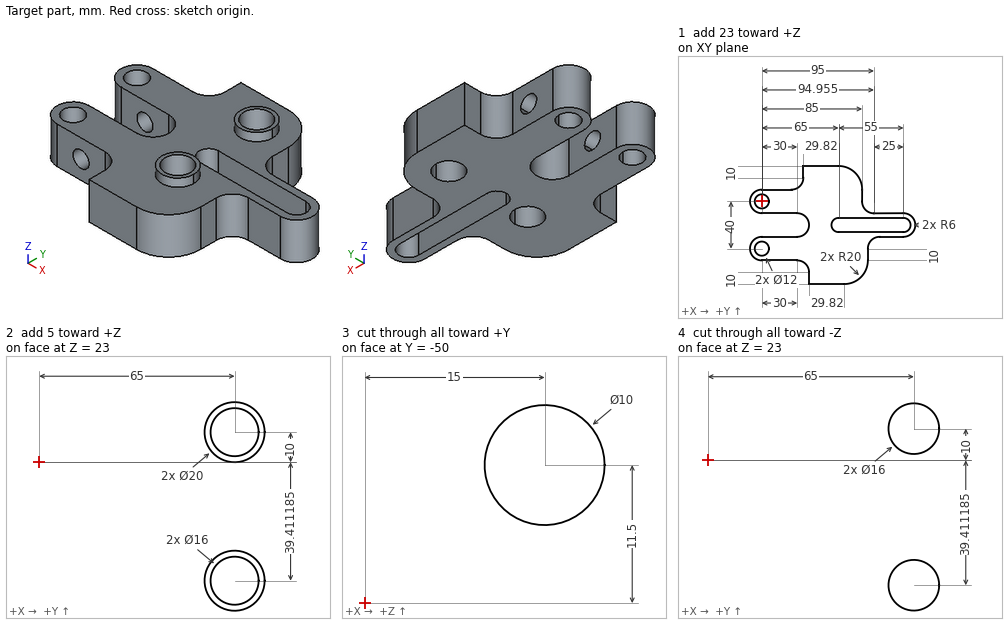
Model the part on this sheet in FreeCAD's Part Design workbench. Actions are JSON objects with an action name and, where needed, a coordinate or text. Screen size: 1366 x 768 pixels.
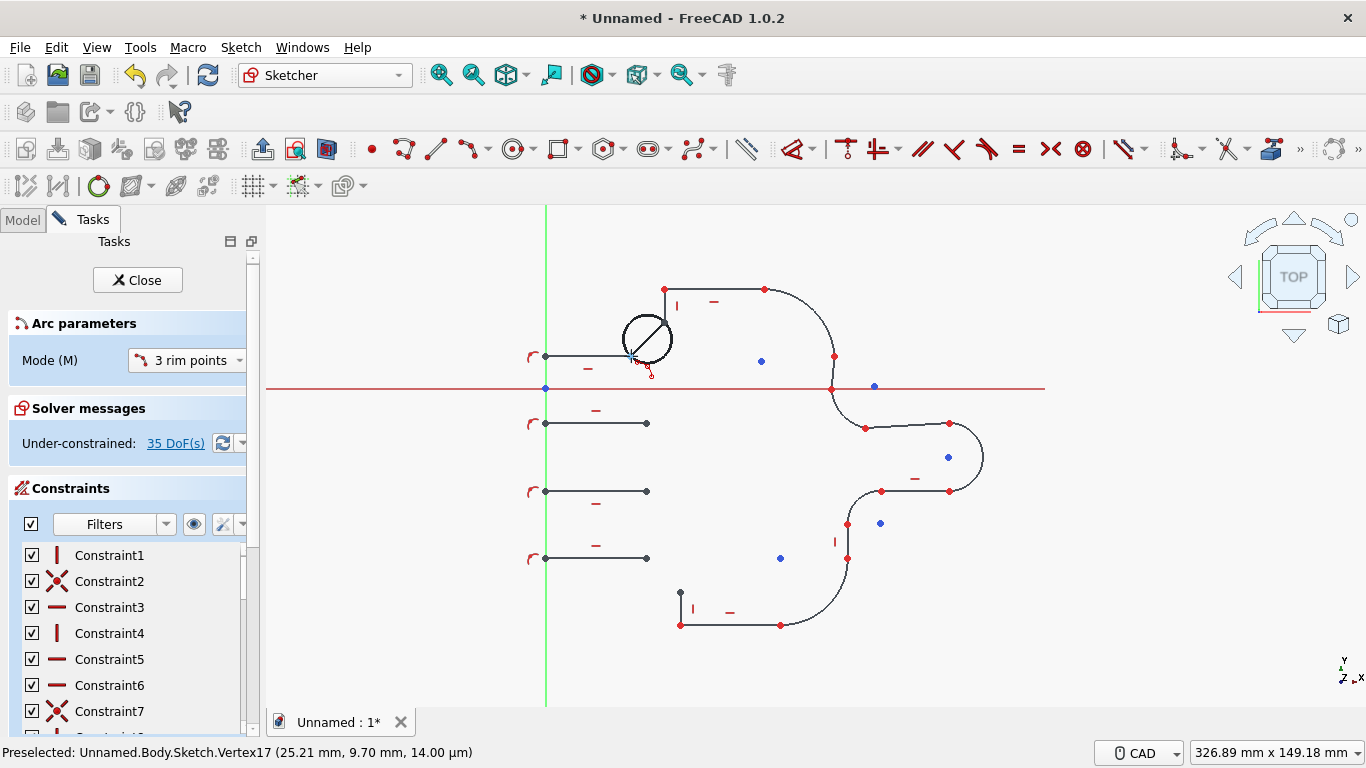
{"action": "scroll", "coordinate": [654, 345], "scroll_direction": "up", "scroll_amount": 3}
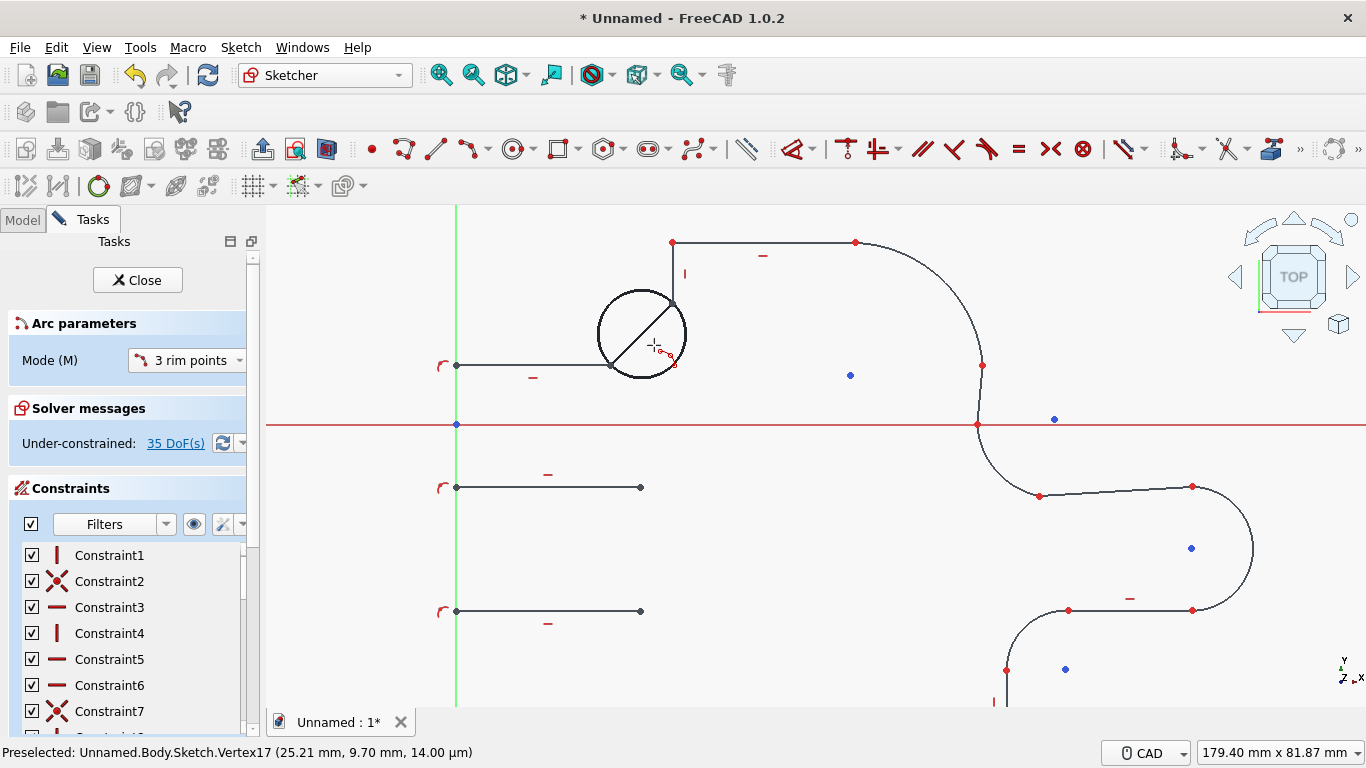
{"action": "left_click", "coordinate": [654, 345]}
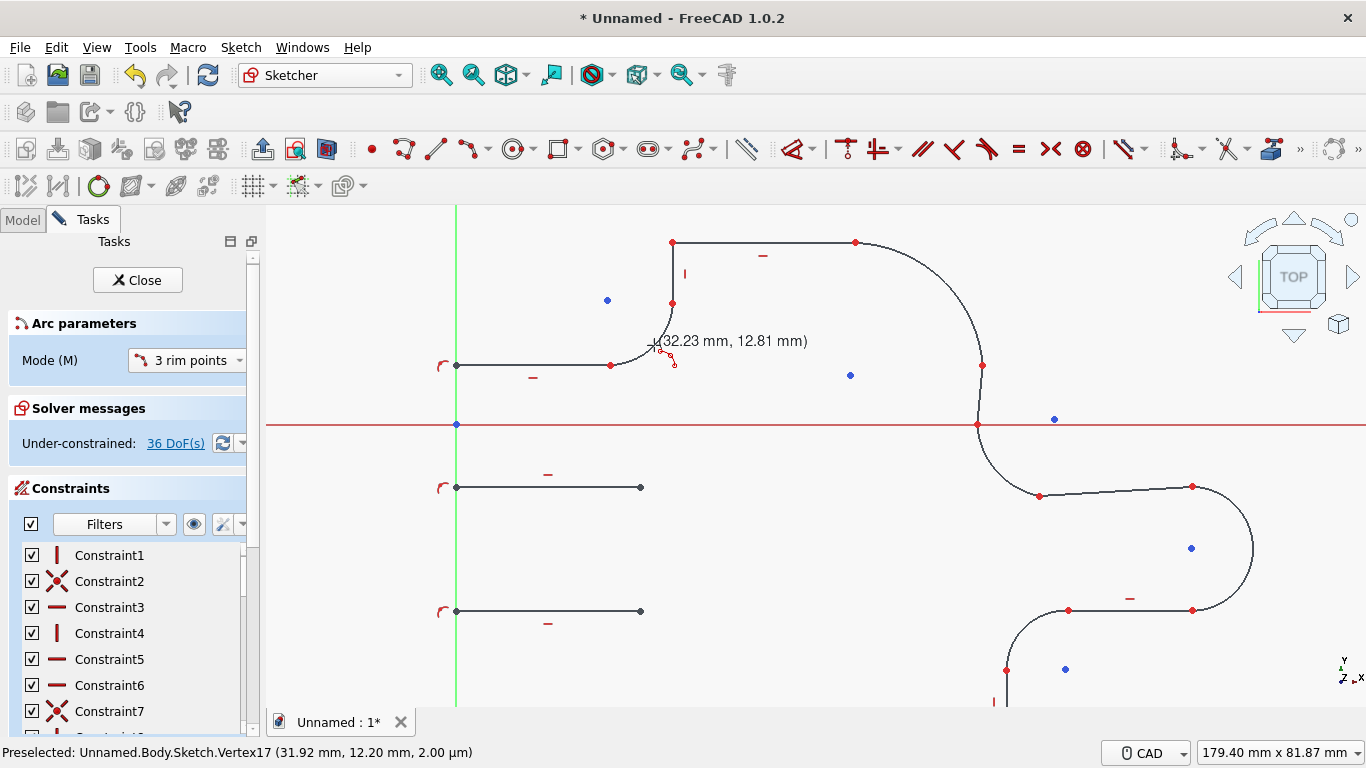
{"action": "left_click", "coordinate": [456, 365]}
{"action": "left_click", "coordinate": [456, 487]}
{"action": "left_click", "coordinate": [407, 389]}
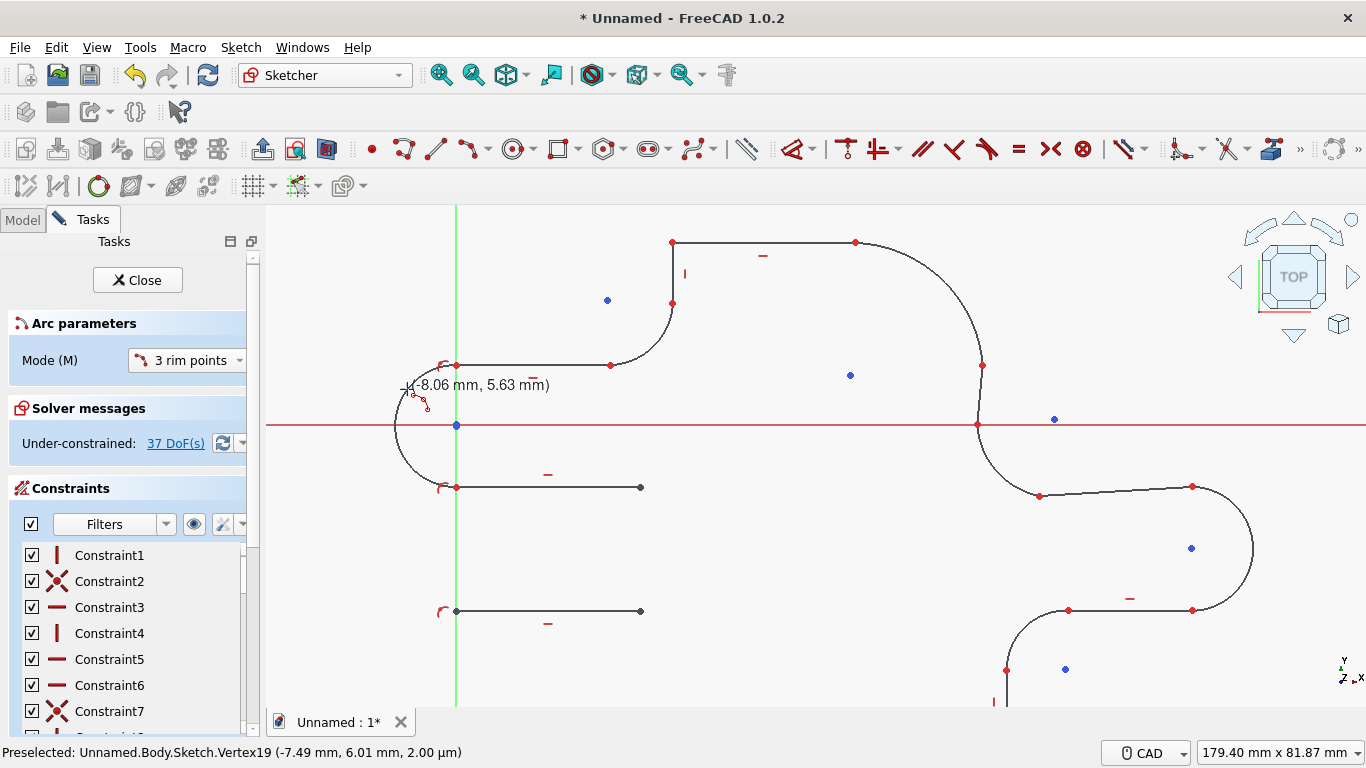
{"action": "left_click", "coordinate": [640, 487]}
{"action": "left_click", "coordinate": [640, 611]}
{"action": "left_click", "coordinate": [702, 547]}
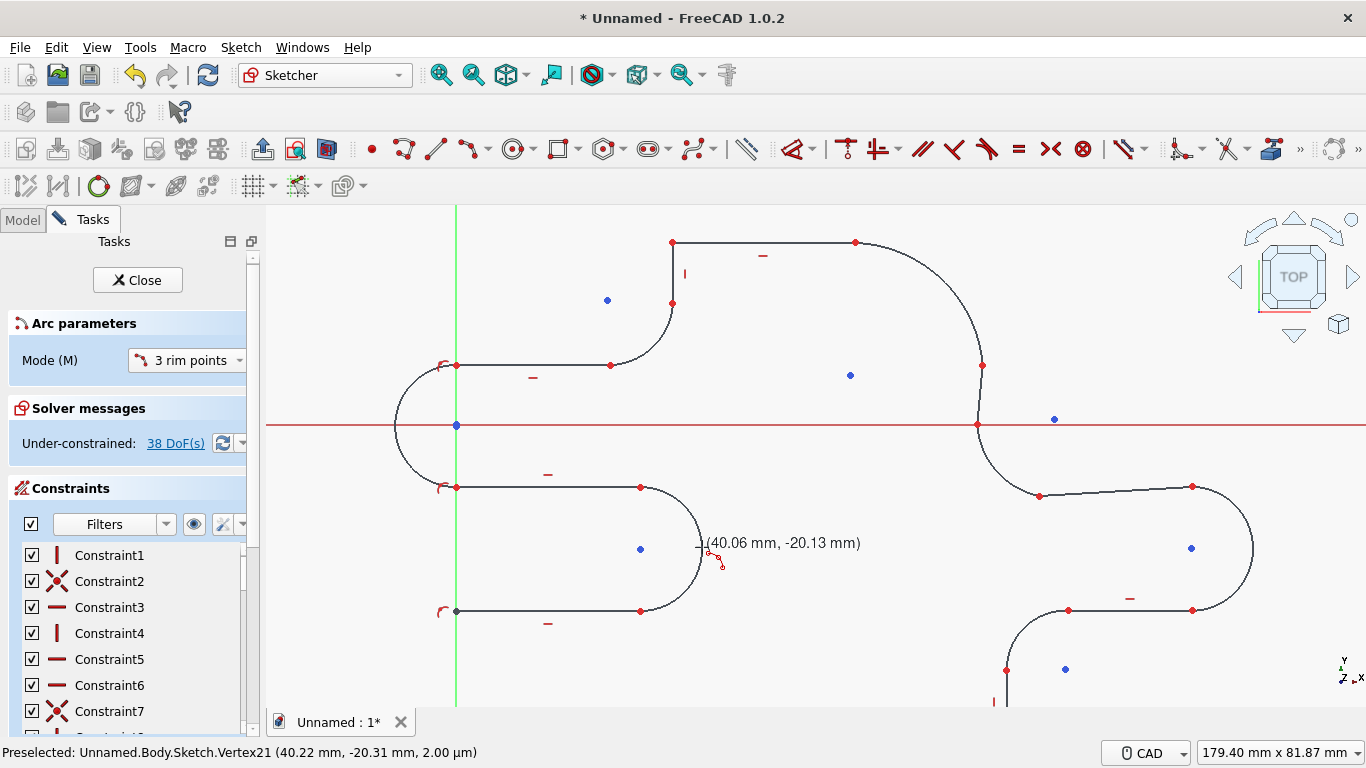
{"action": "left_click", "coordinate": [456, 611]}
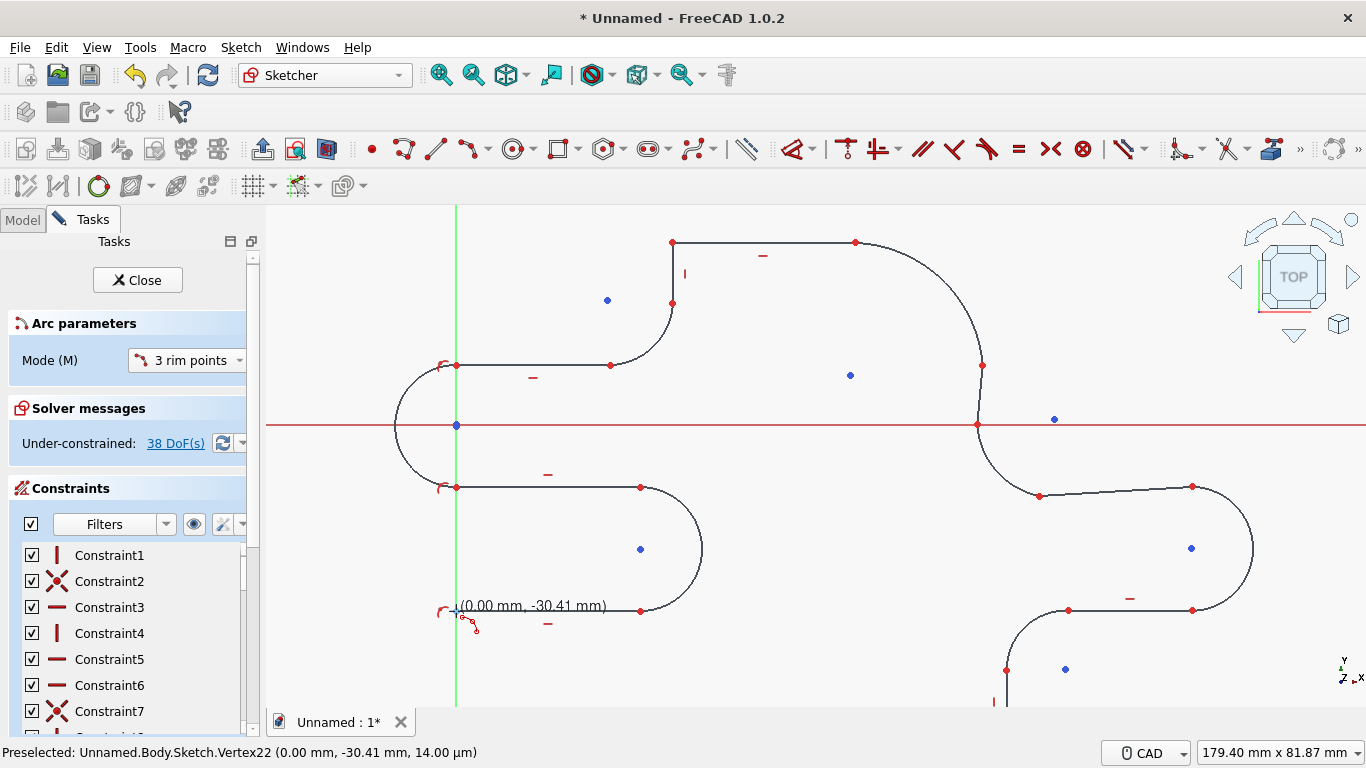
{"action": "scroll", "coordinate": [654, 345], "scroll_direction": "down", "scroll_amount": 3}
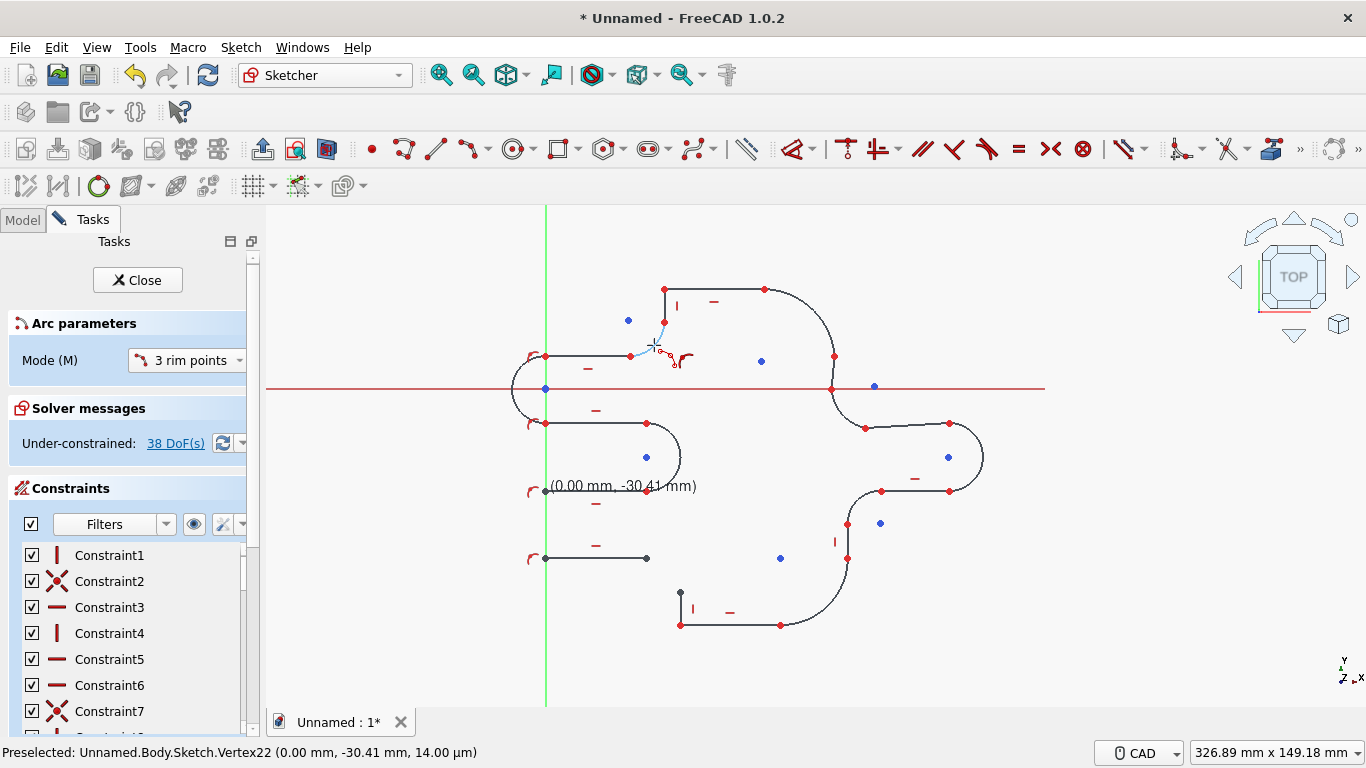
{"action": "left_click", "coordinate": [546, 558]}
{"action": "left_click", "coordinate": [512, 523]}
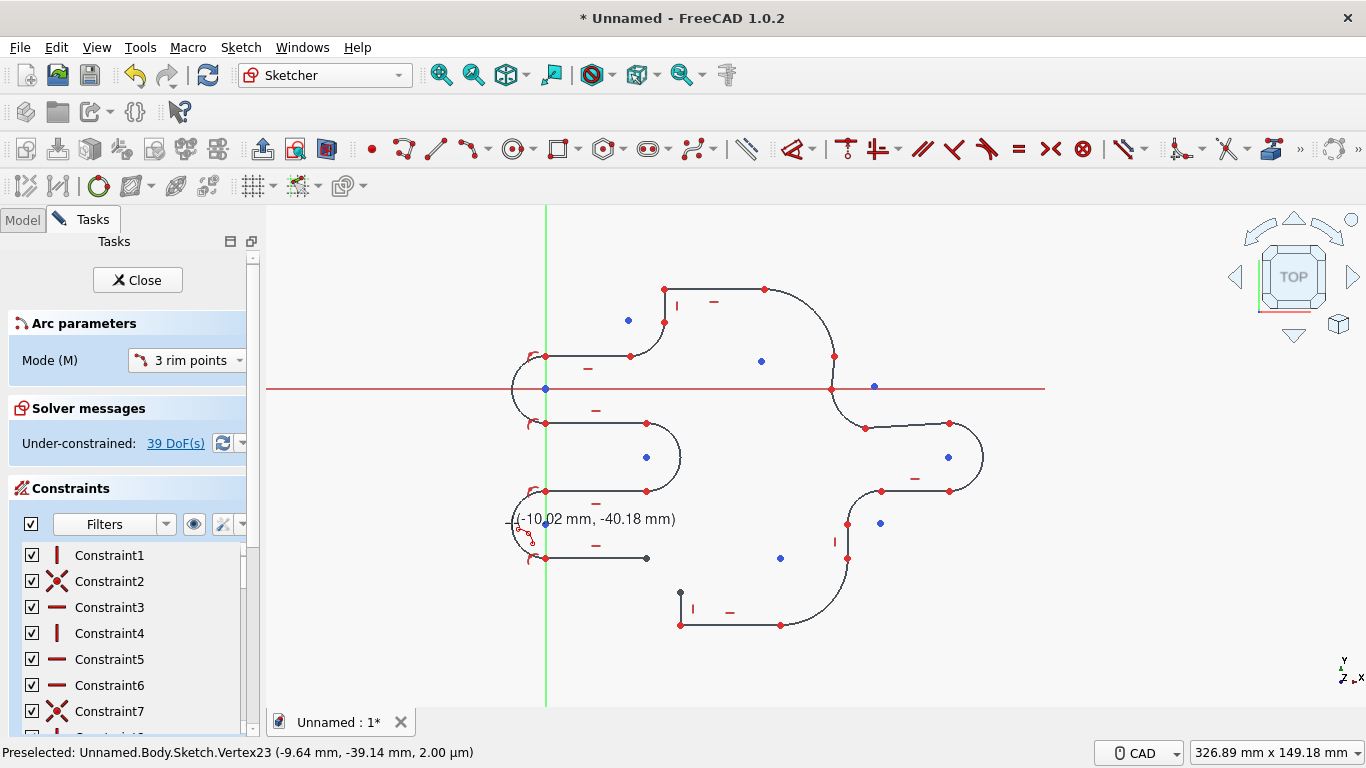
{"action": "left_click", "coordinate": [647, 558]}
{"action": "left_click", "coordinate": [681, 592]}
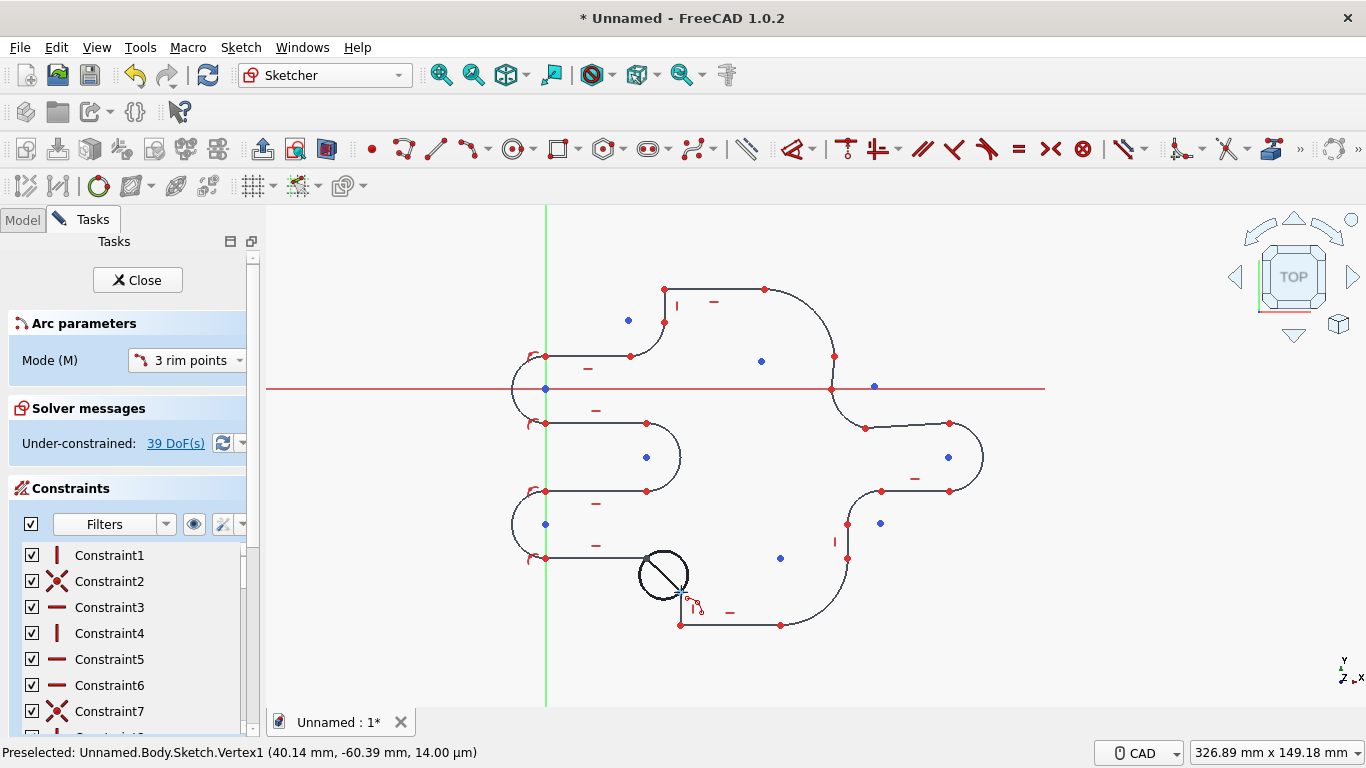
{"action": "scroll", "coordinate": [670, 567], "scroll_direction": "up", "scroll_amount": 3}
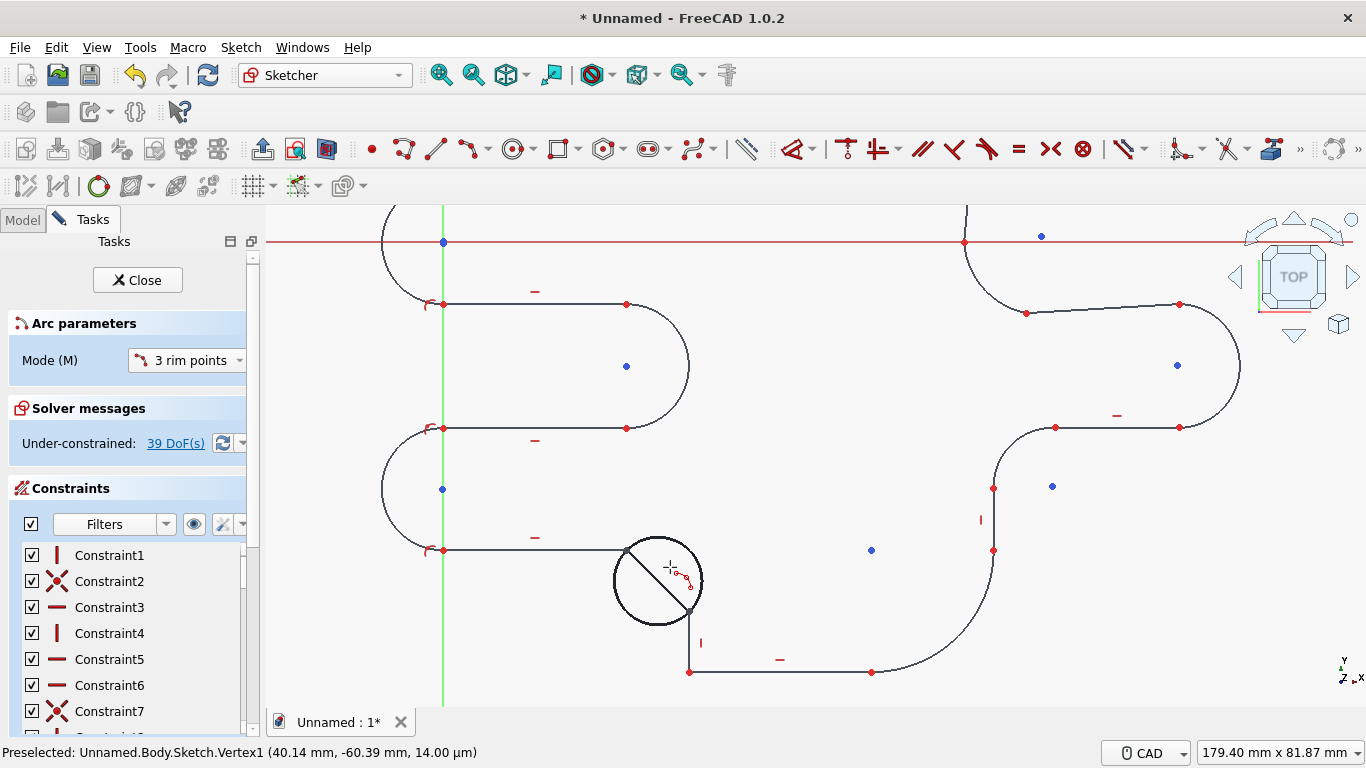
{"action": "left_click", "coordinate": [671, 566]}